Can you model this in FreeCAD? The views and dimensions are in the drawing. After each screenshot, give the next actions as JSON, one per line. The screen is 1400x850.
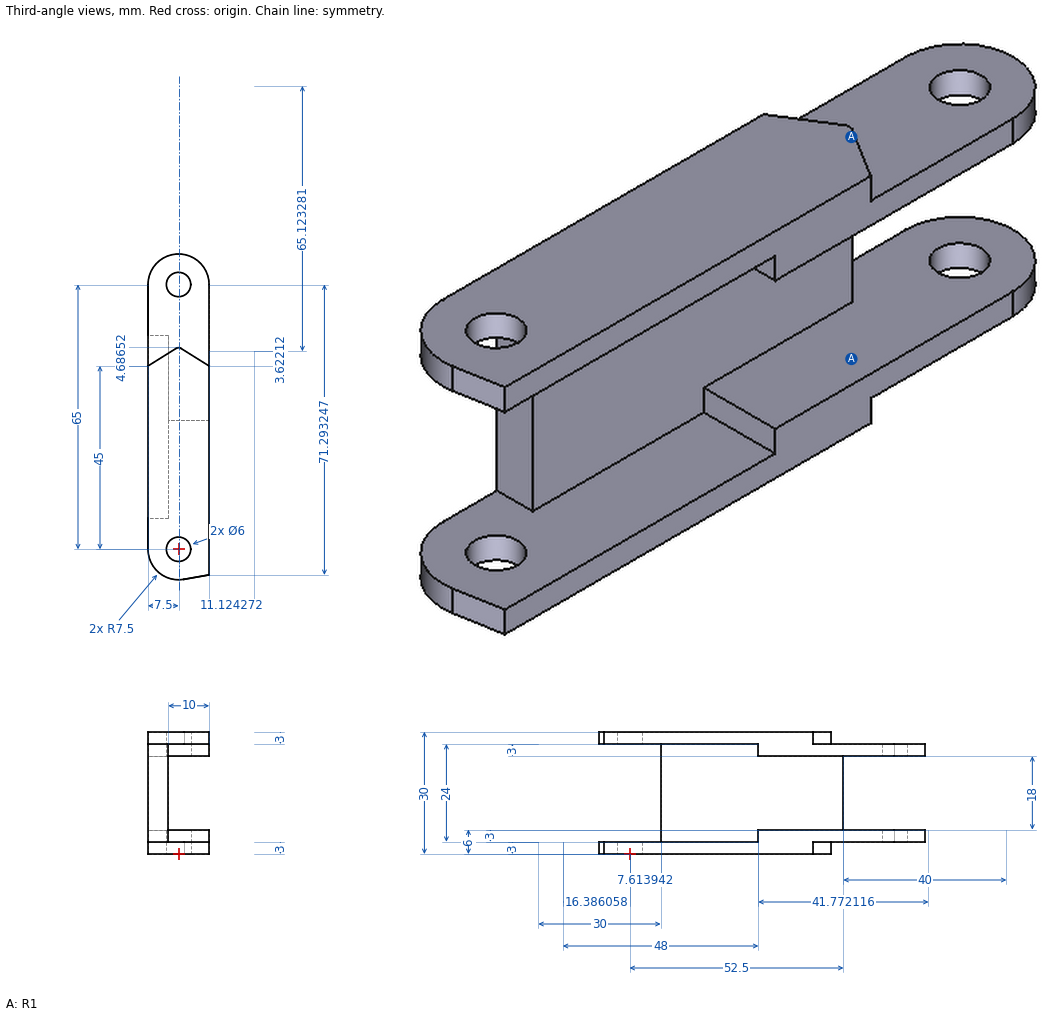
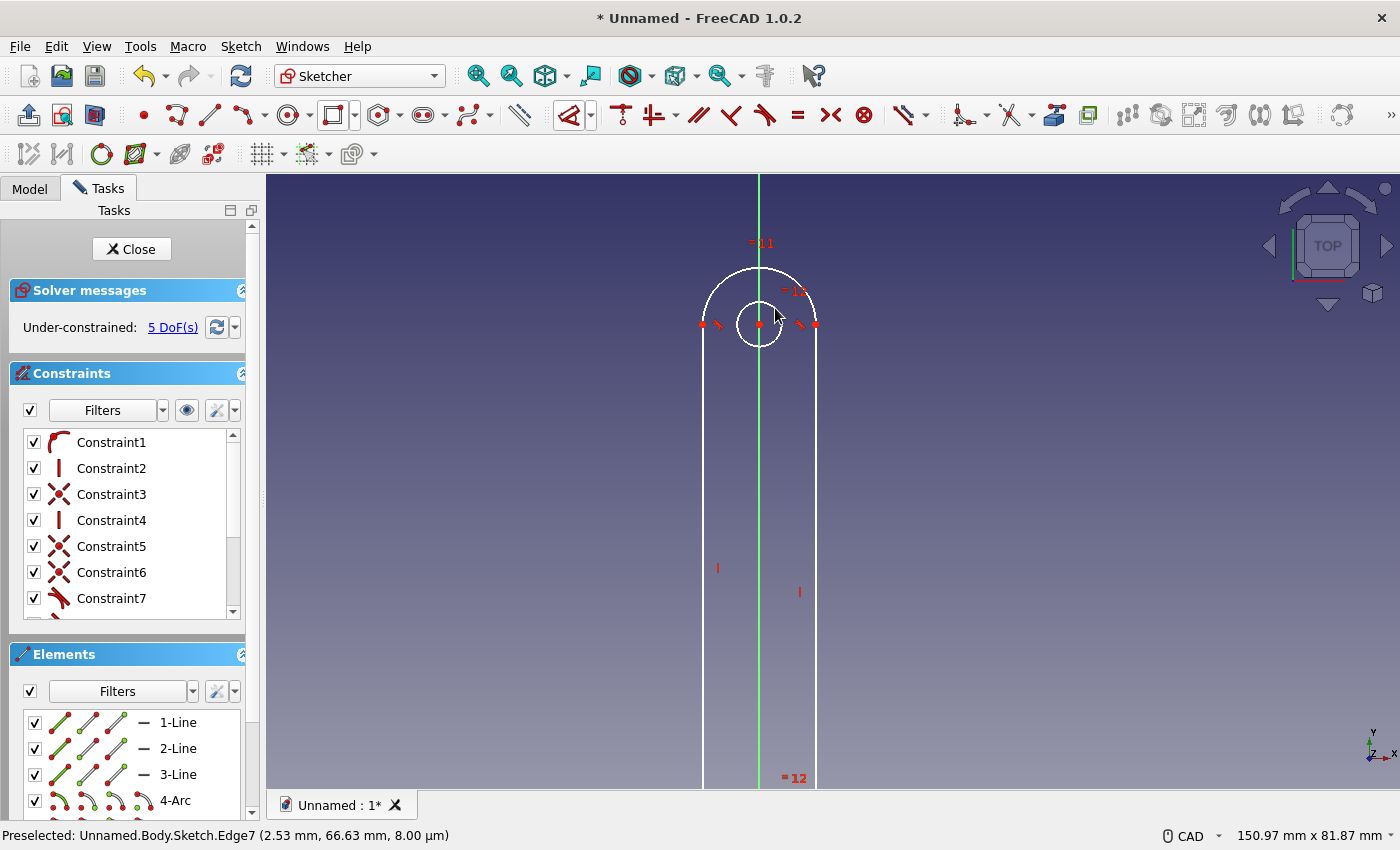
{"action": "scroll", "coordinate": [776, 308], "scroll_direction": "down", "scroll_amount": 2}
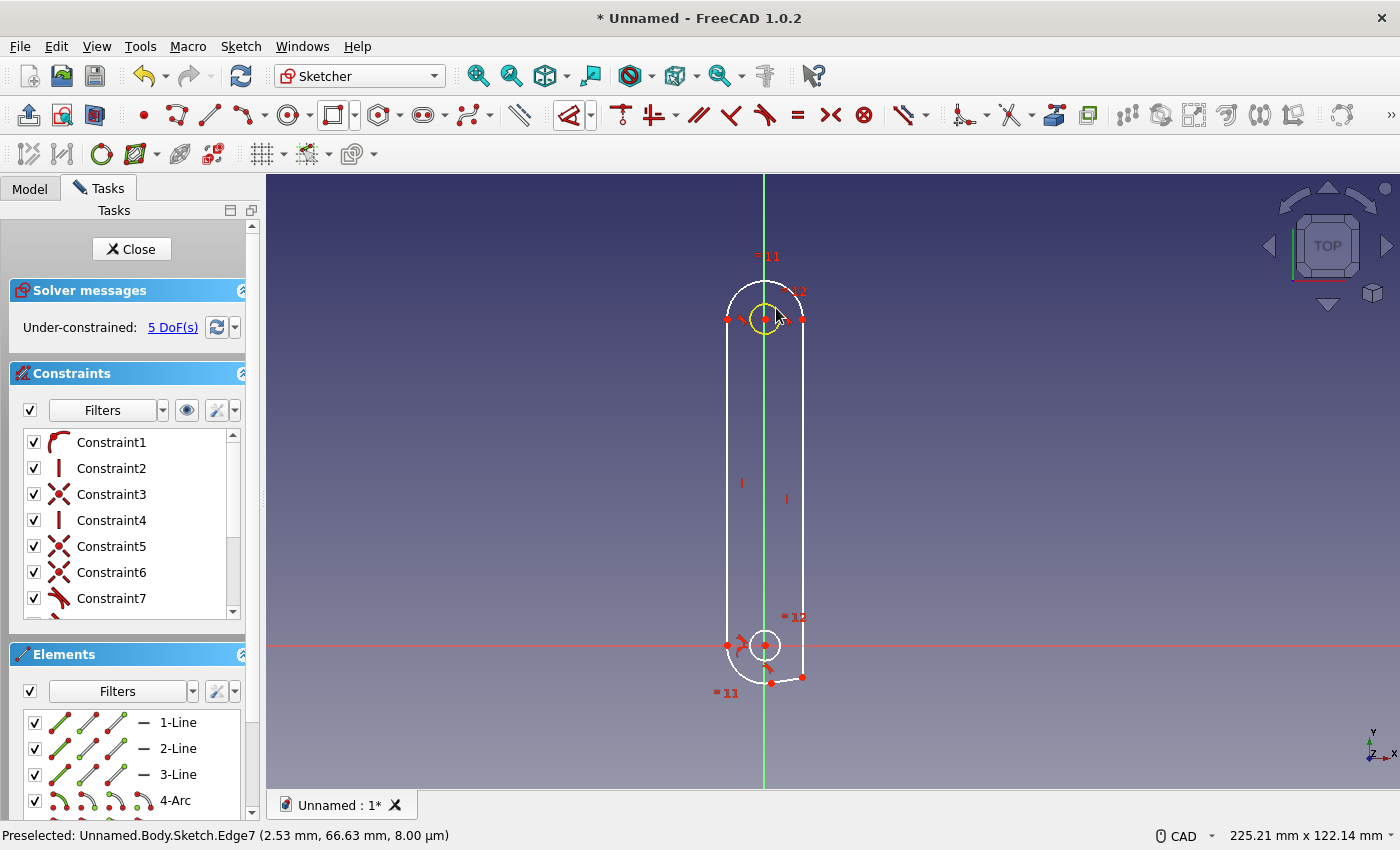
{"action": "left_click", "coordinate": [765, 646]}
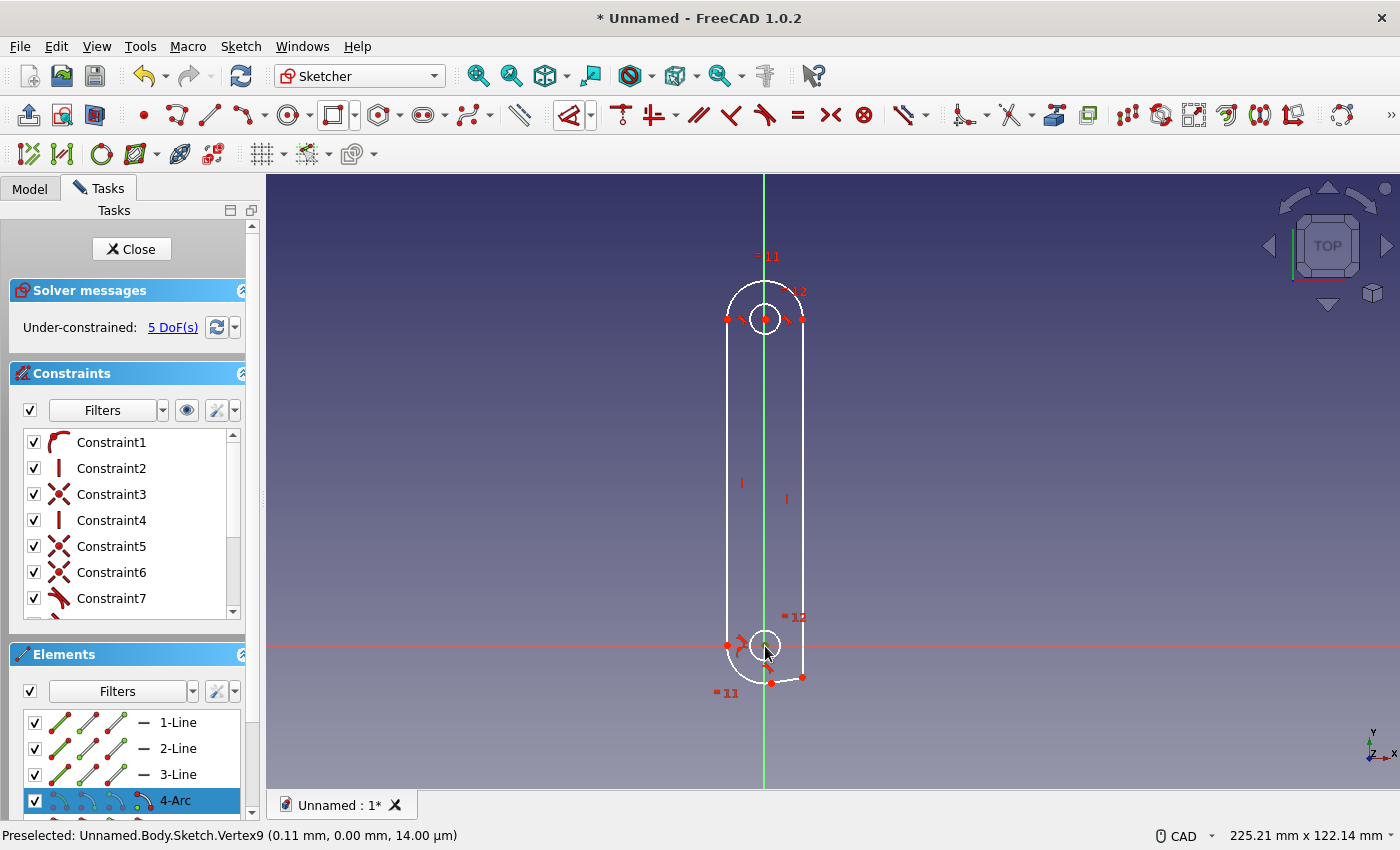
{"action": "left_click", "coordinate": [764, 721]}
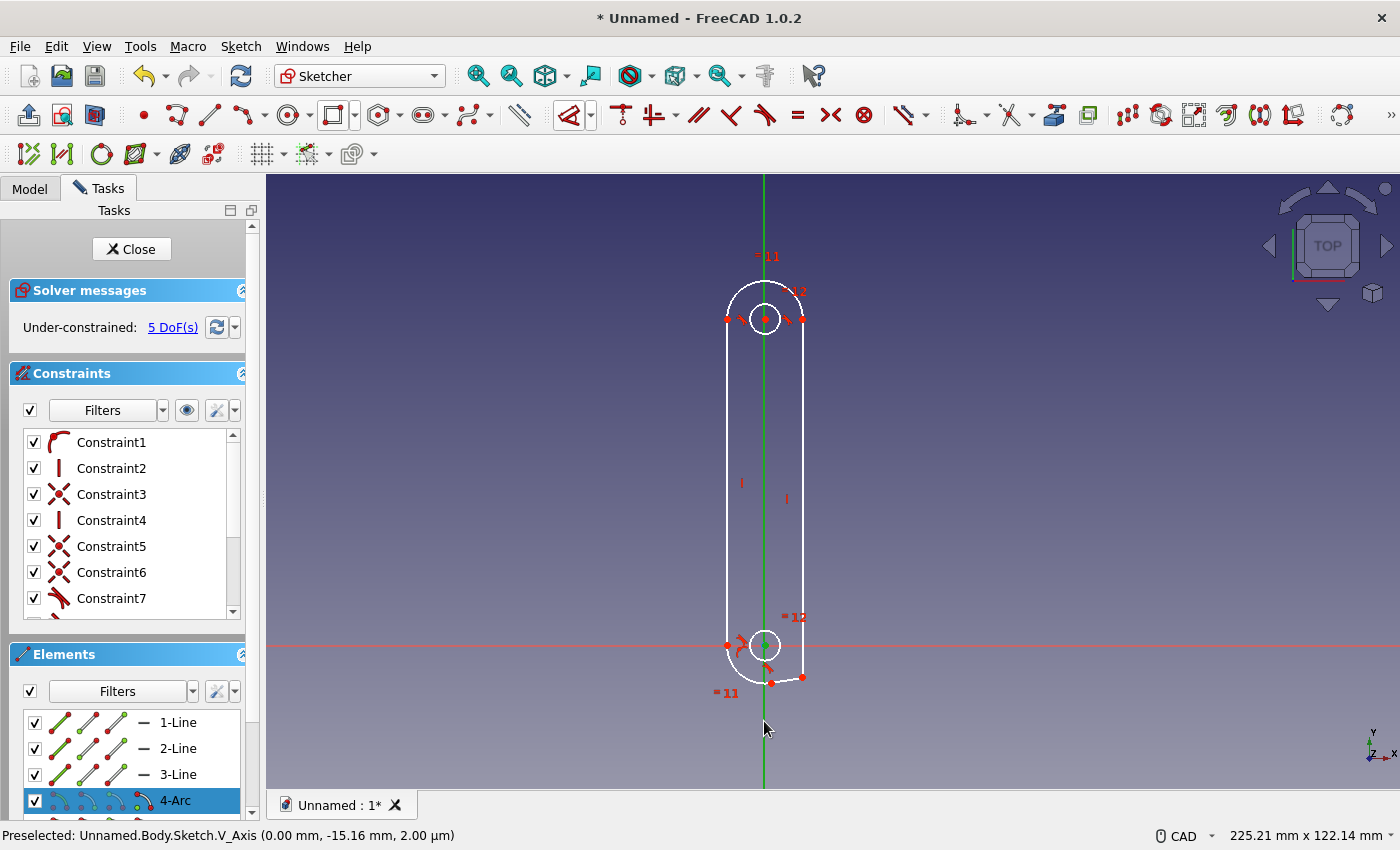
{"action": "left_click", "coordinate": [621, 116]}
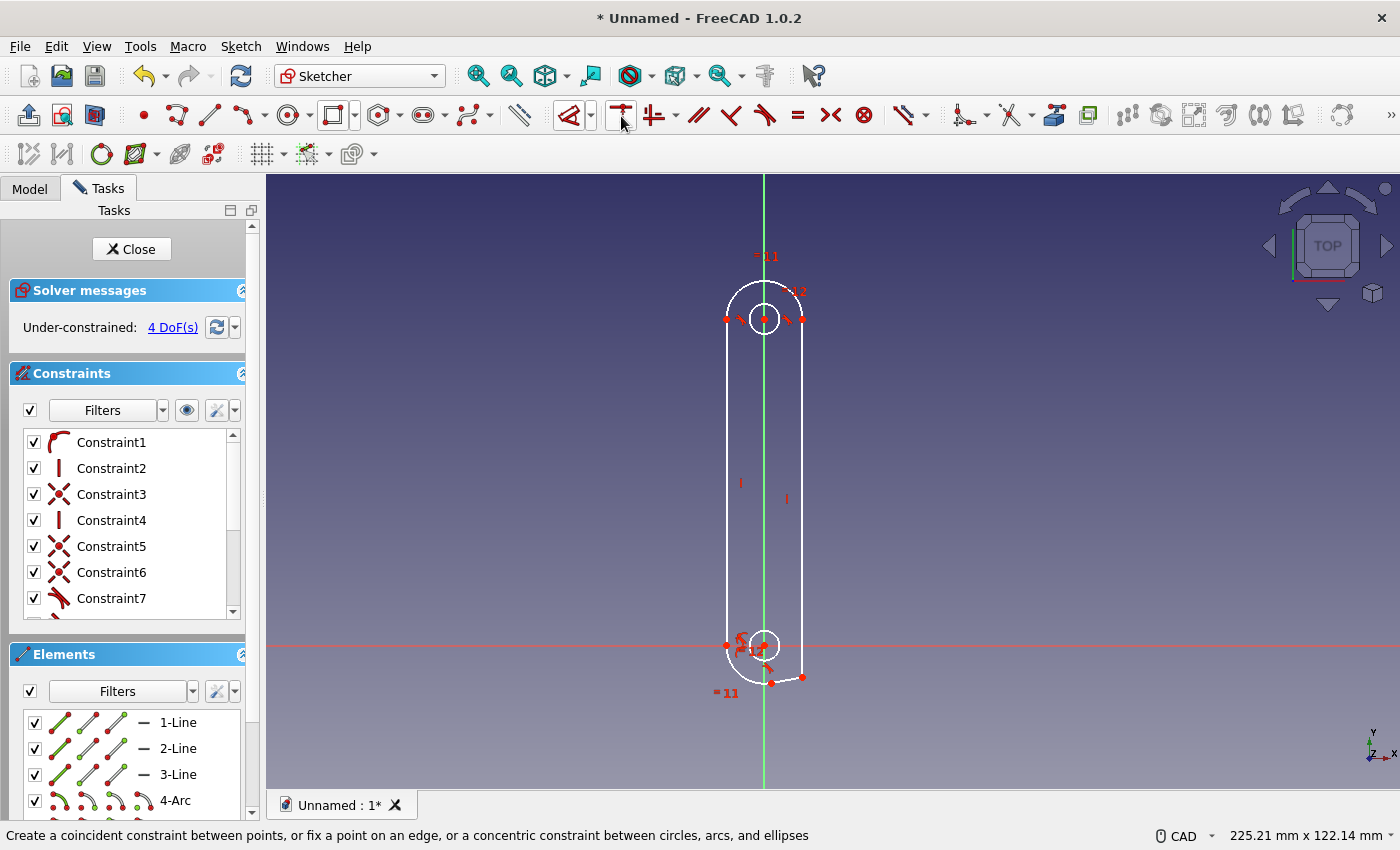
{"action": "left_click", "coordinate": [732, 665]}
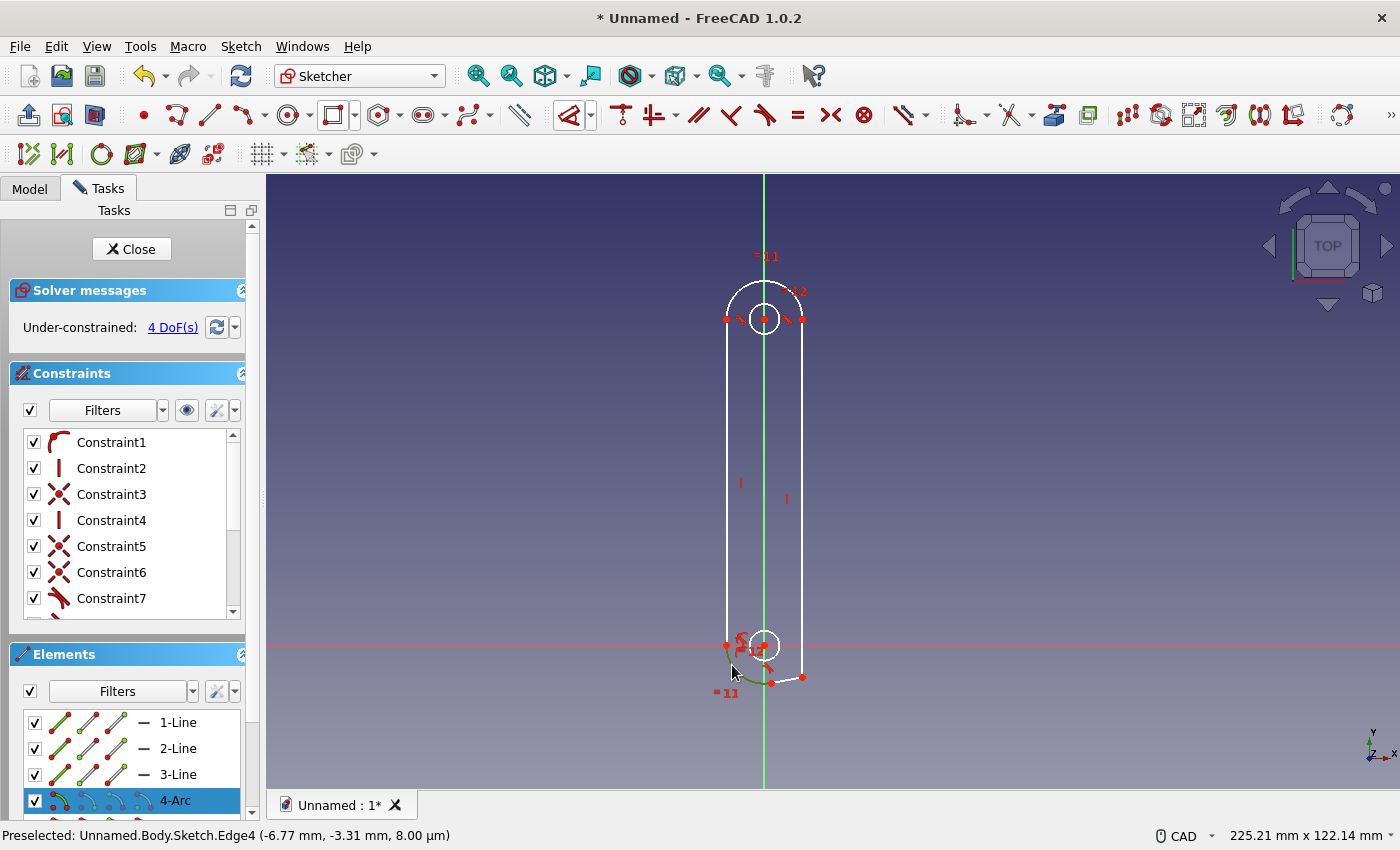
{"action": "key", "text": "k r"}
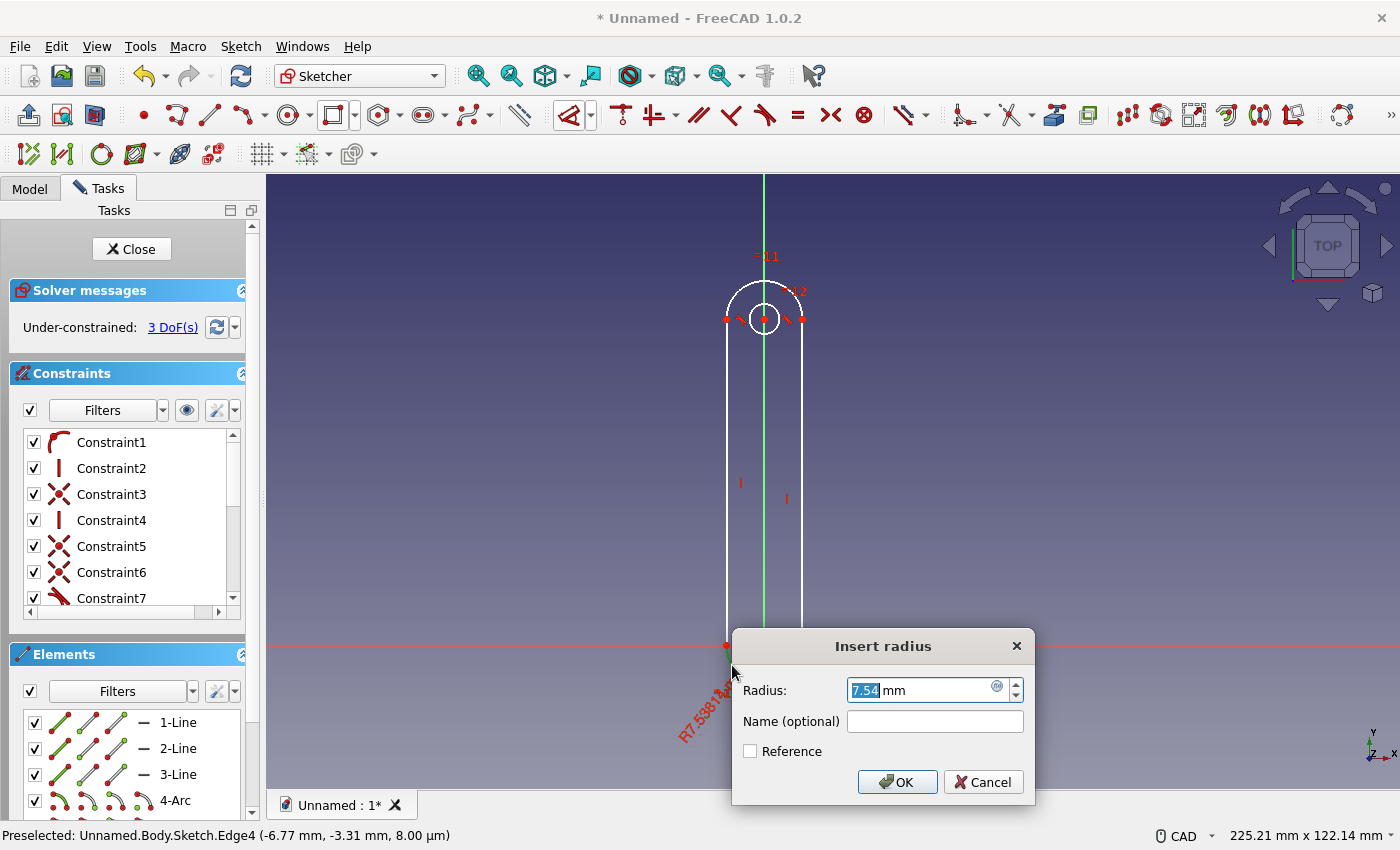
{"action": "type", "text": "7.5"}
{"action": "key", "text": "Return"}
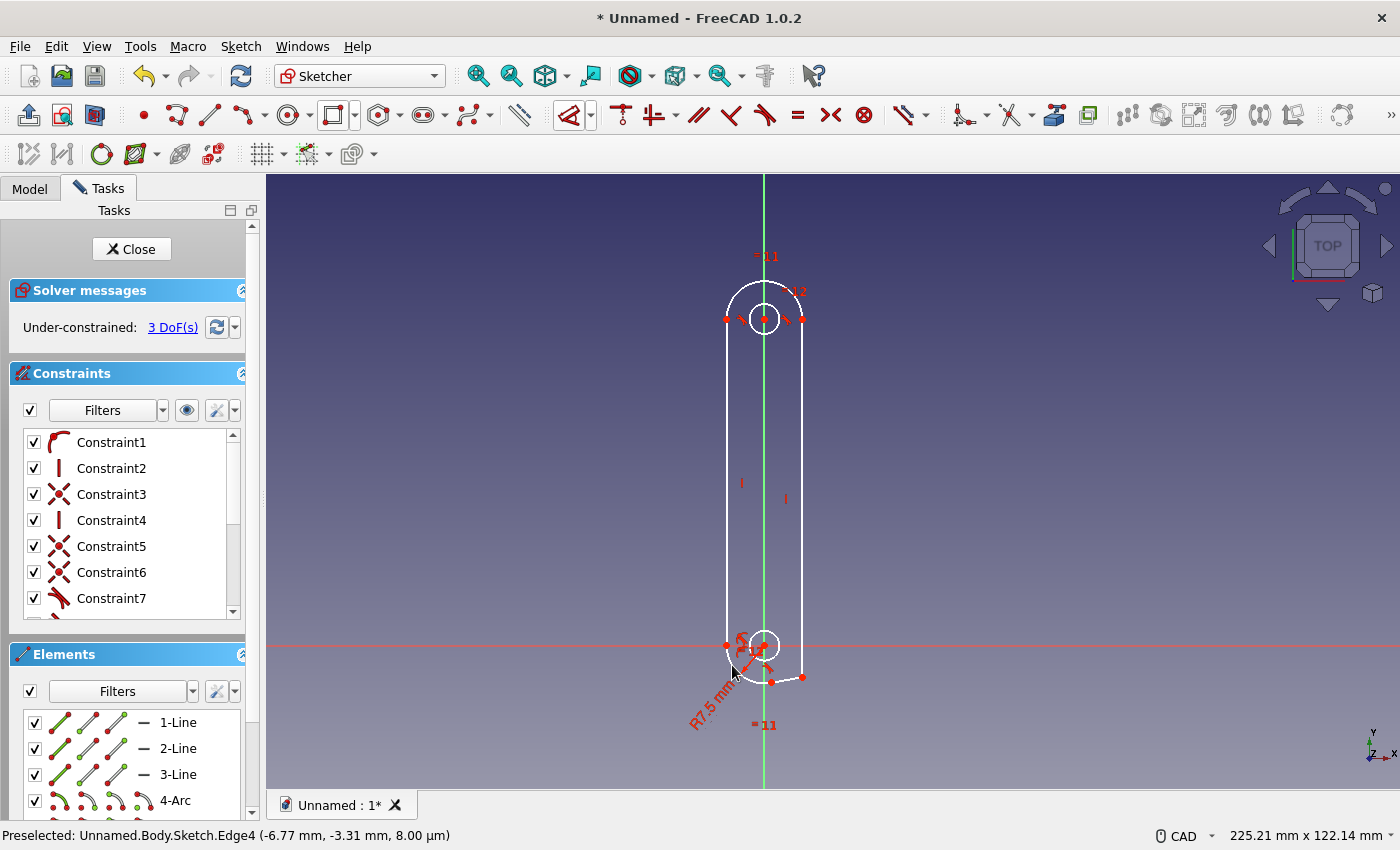
{"action": "scroll", "coordinate": [775, 635], "scroll_direction": "up", "scroll_amount": 2}